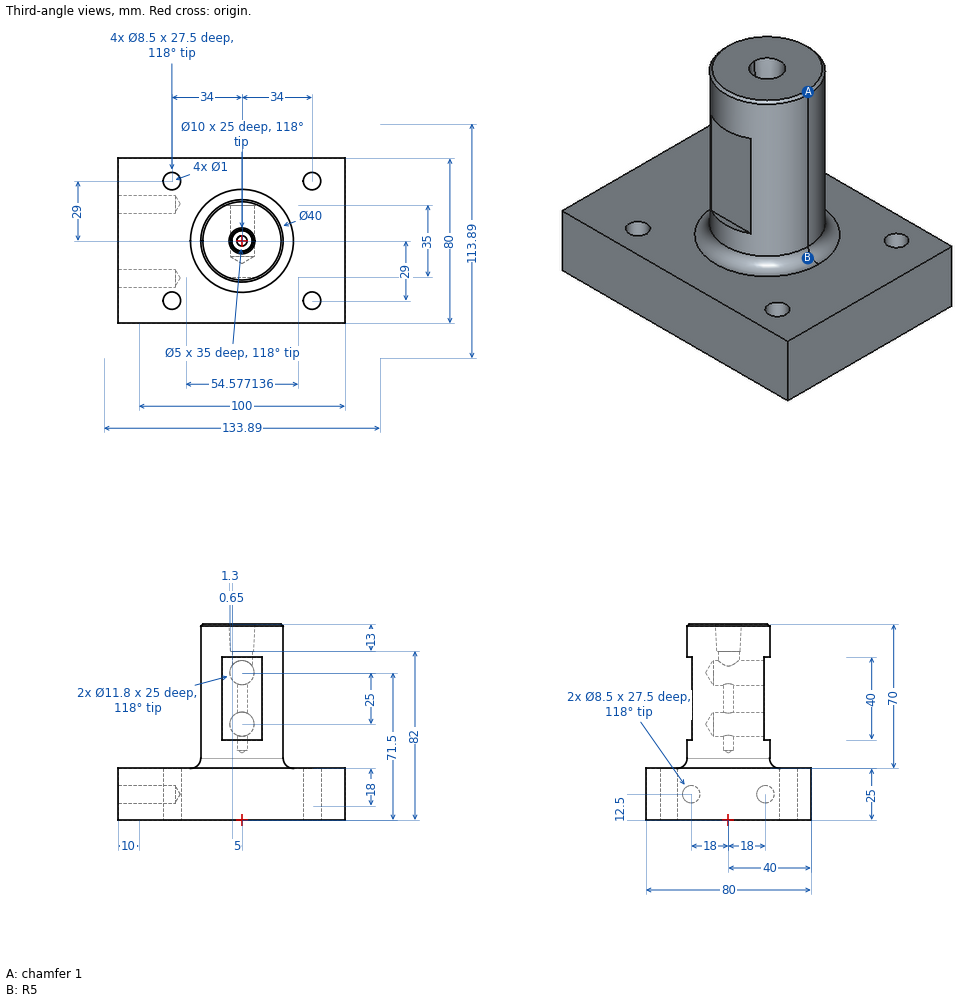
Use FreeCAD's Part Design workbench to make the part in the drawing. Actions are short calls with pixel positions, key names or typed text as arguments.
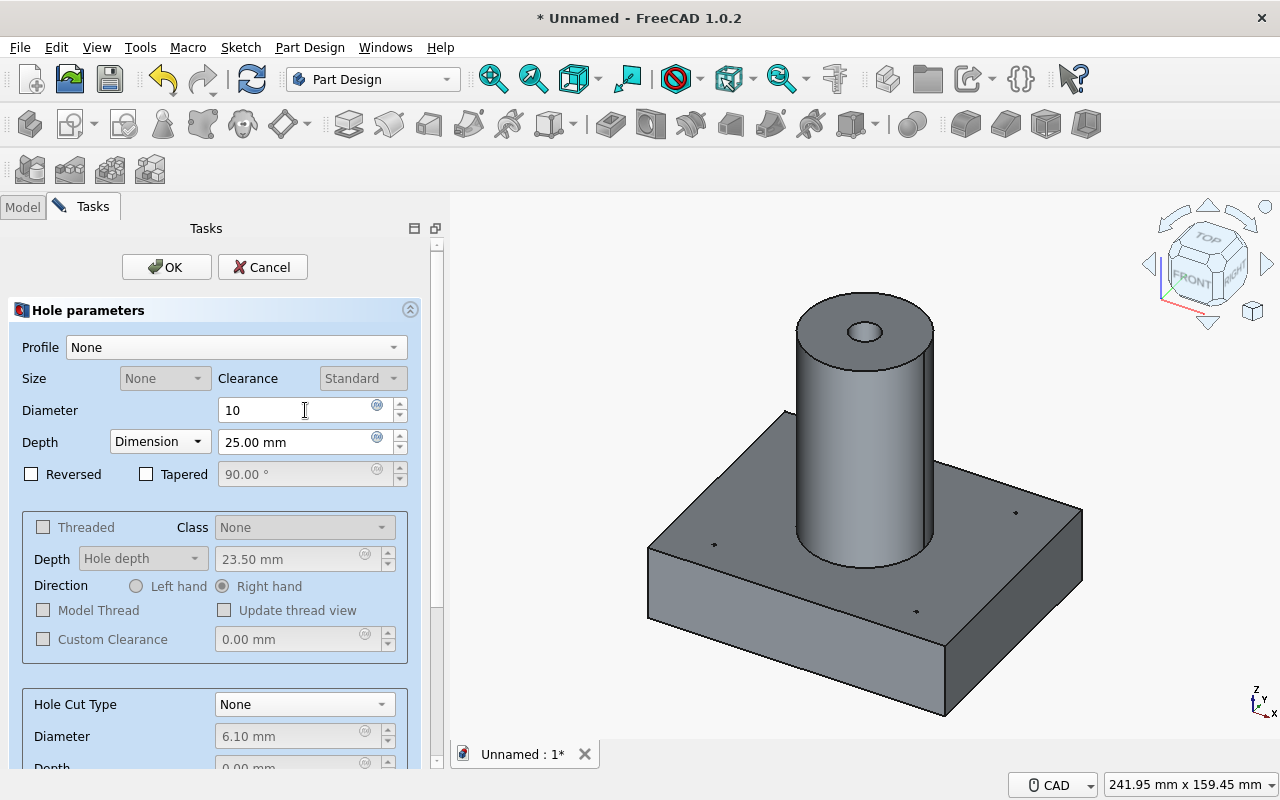
triple_click(305, 442)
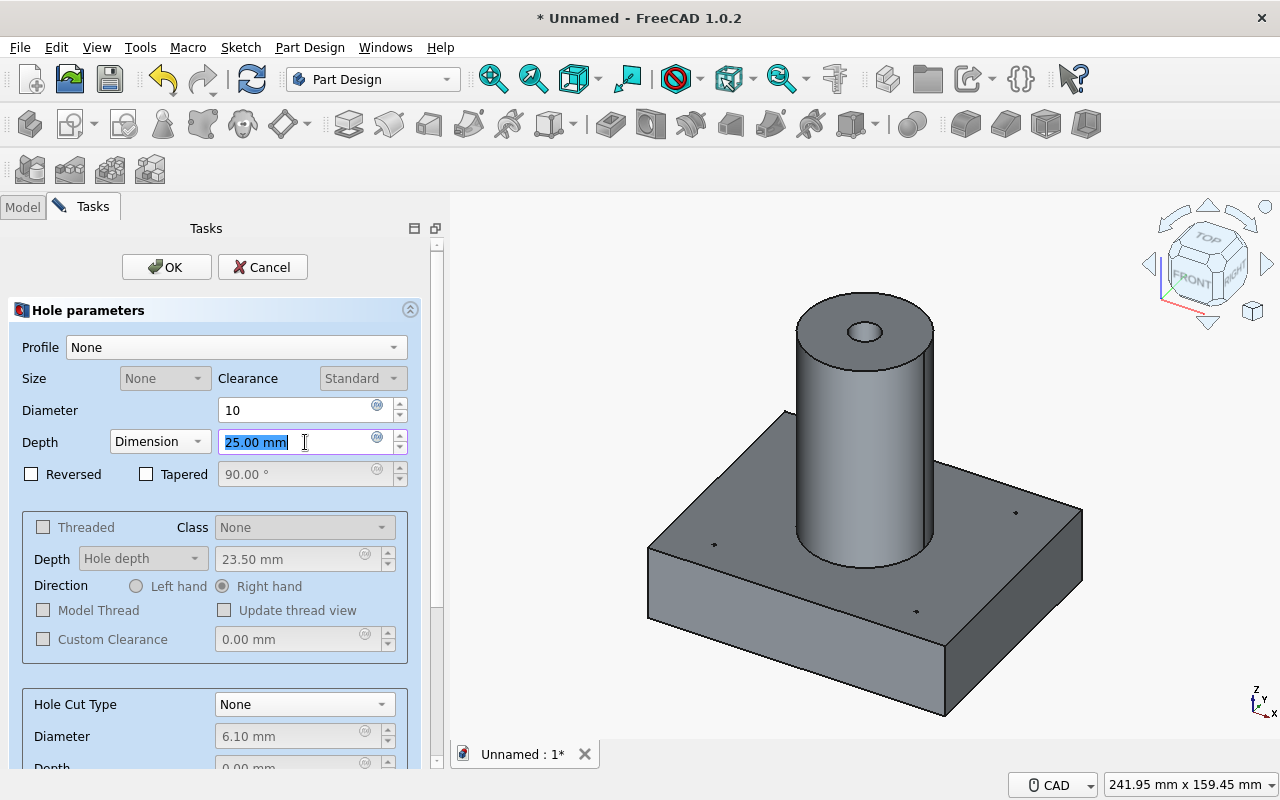
text(25)
key(Tab)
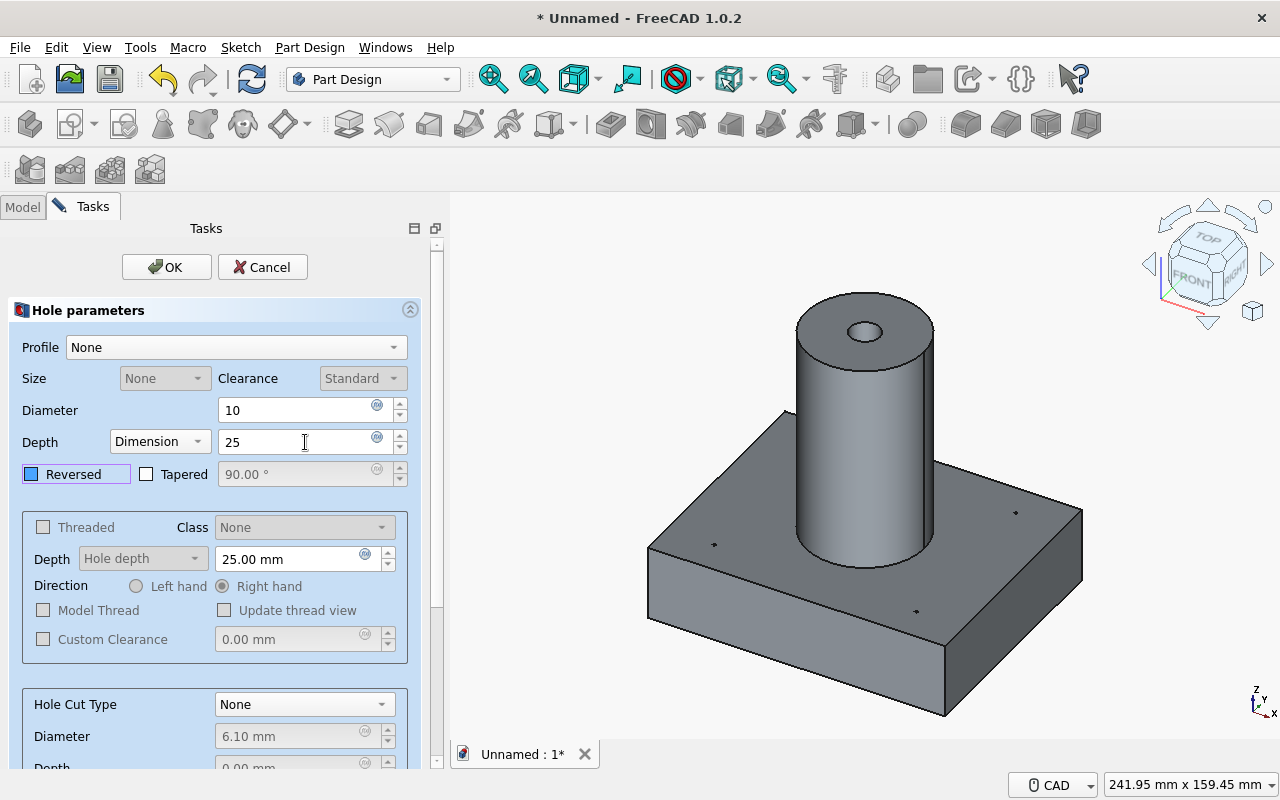
click(167, 267)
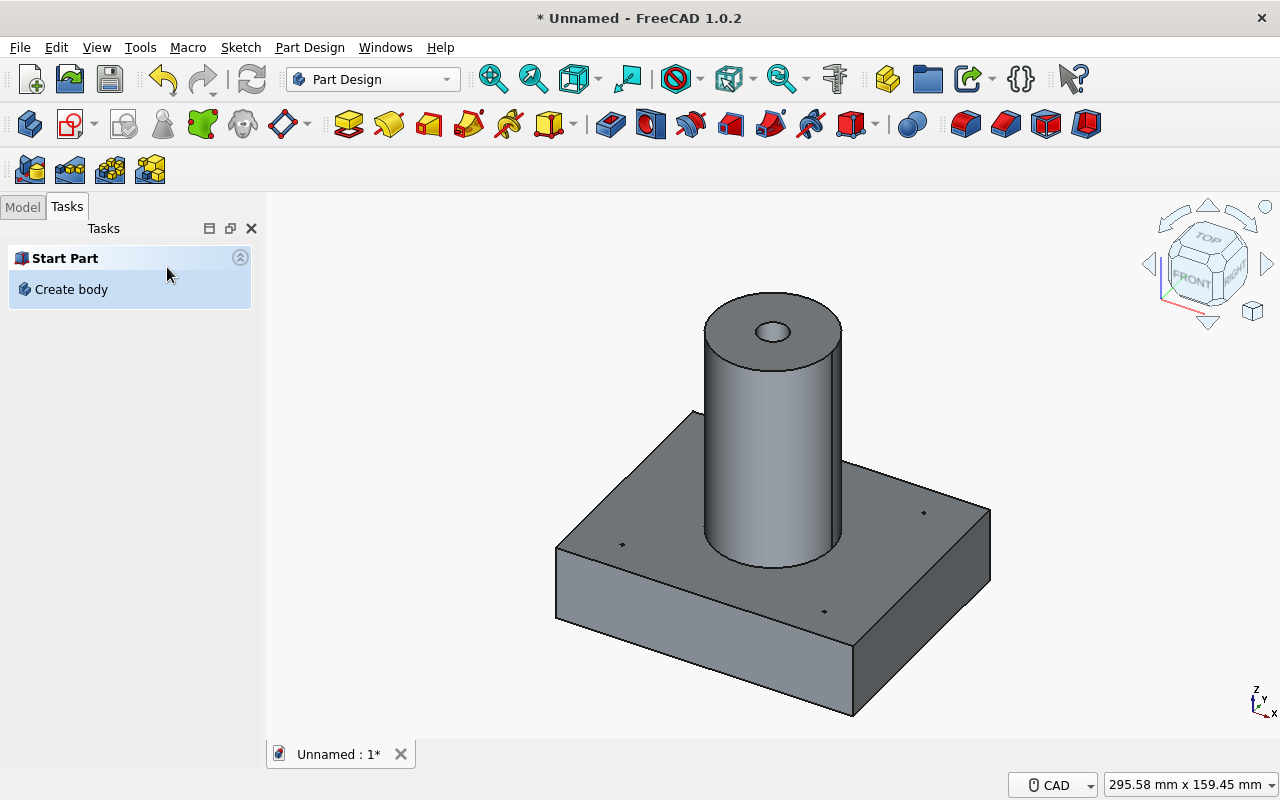
click(70, 124)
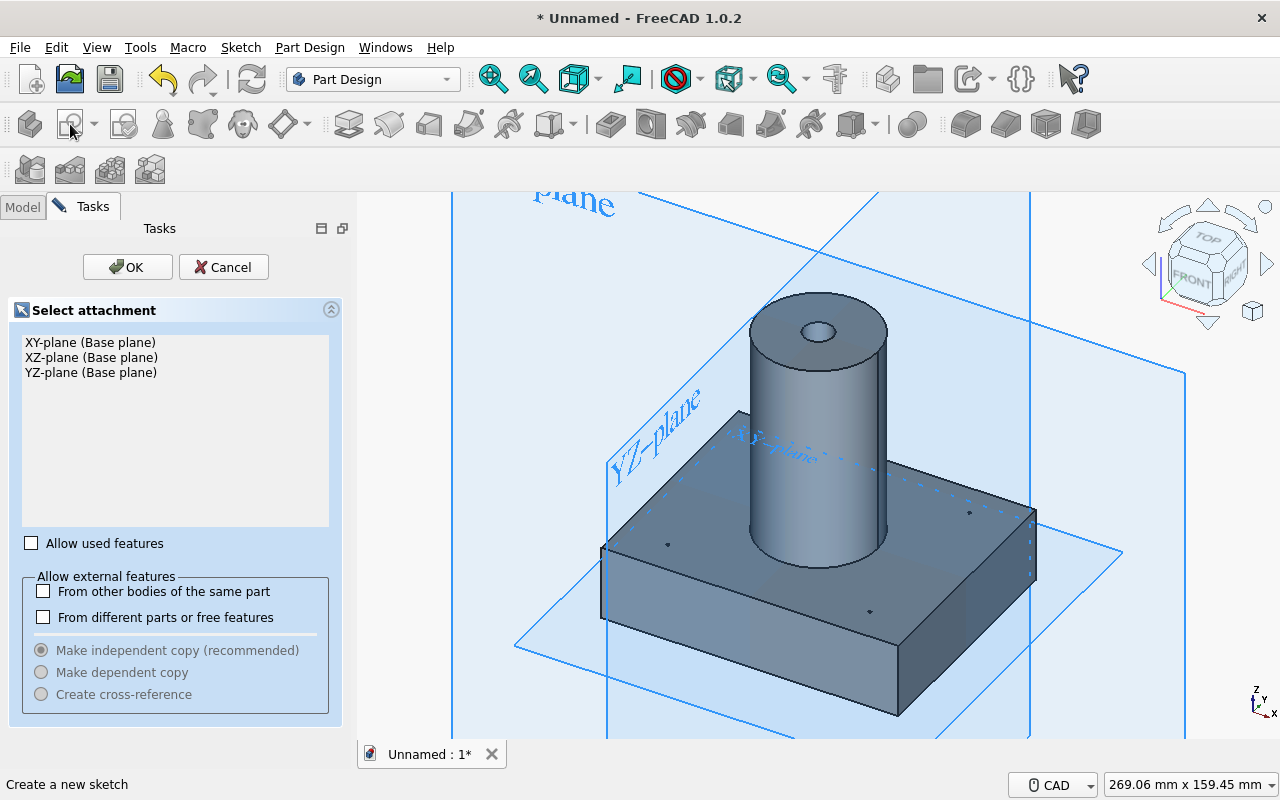
click(82, 358)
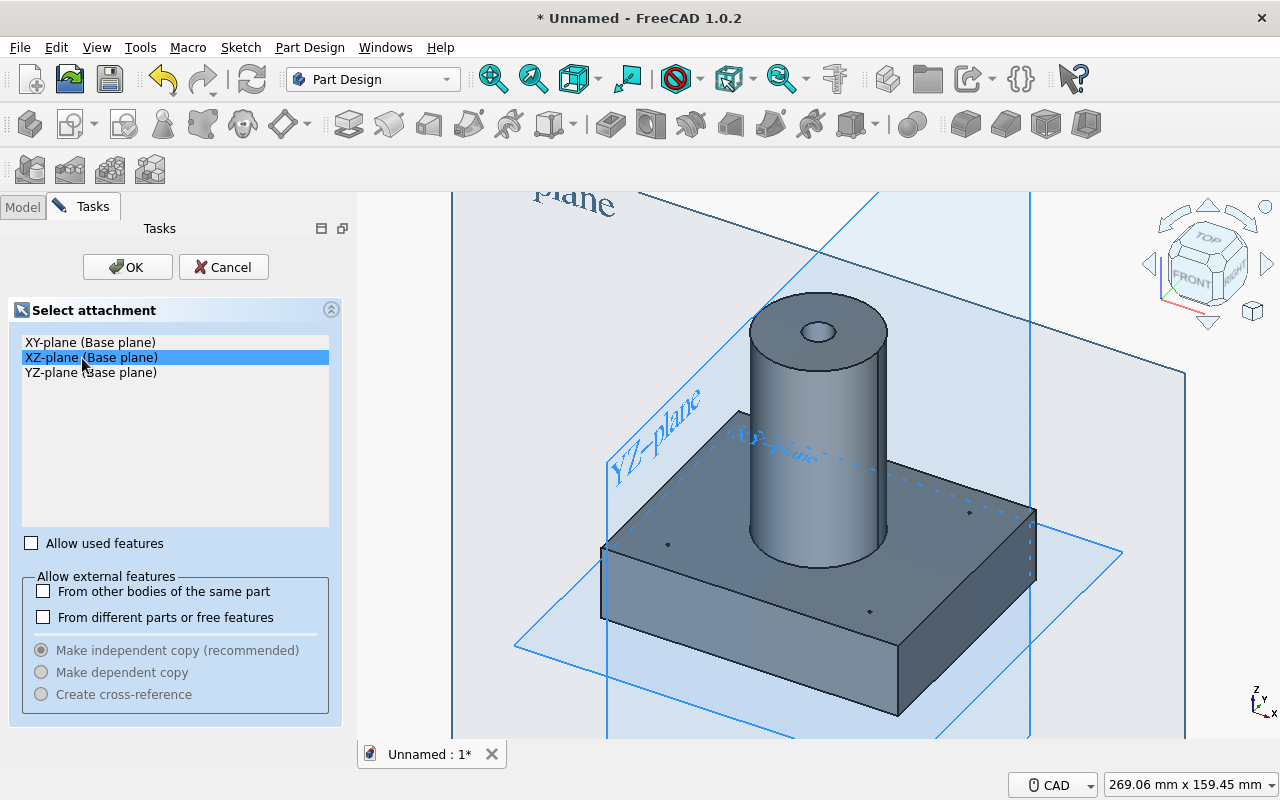
click(128, 267)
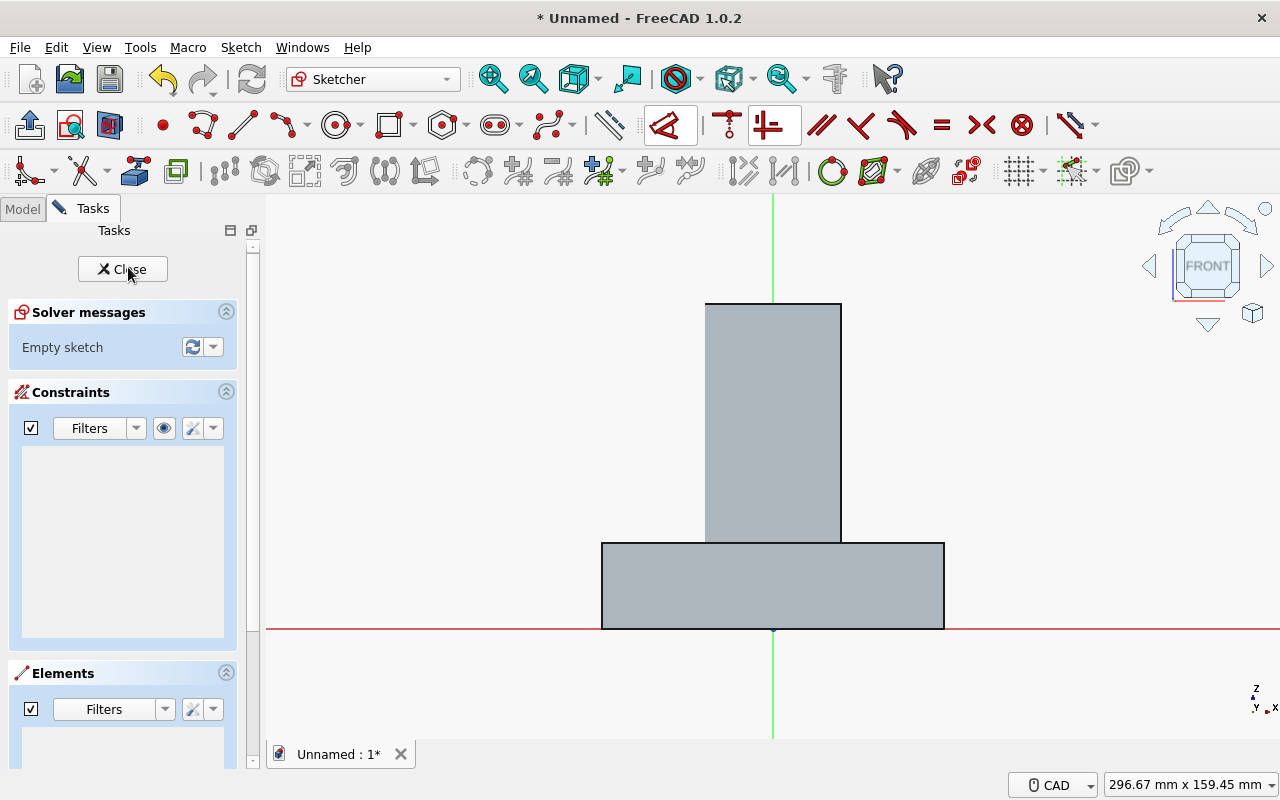
click(110, 126)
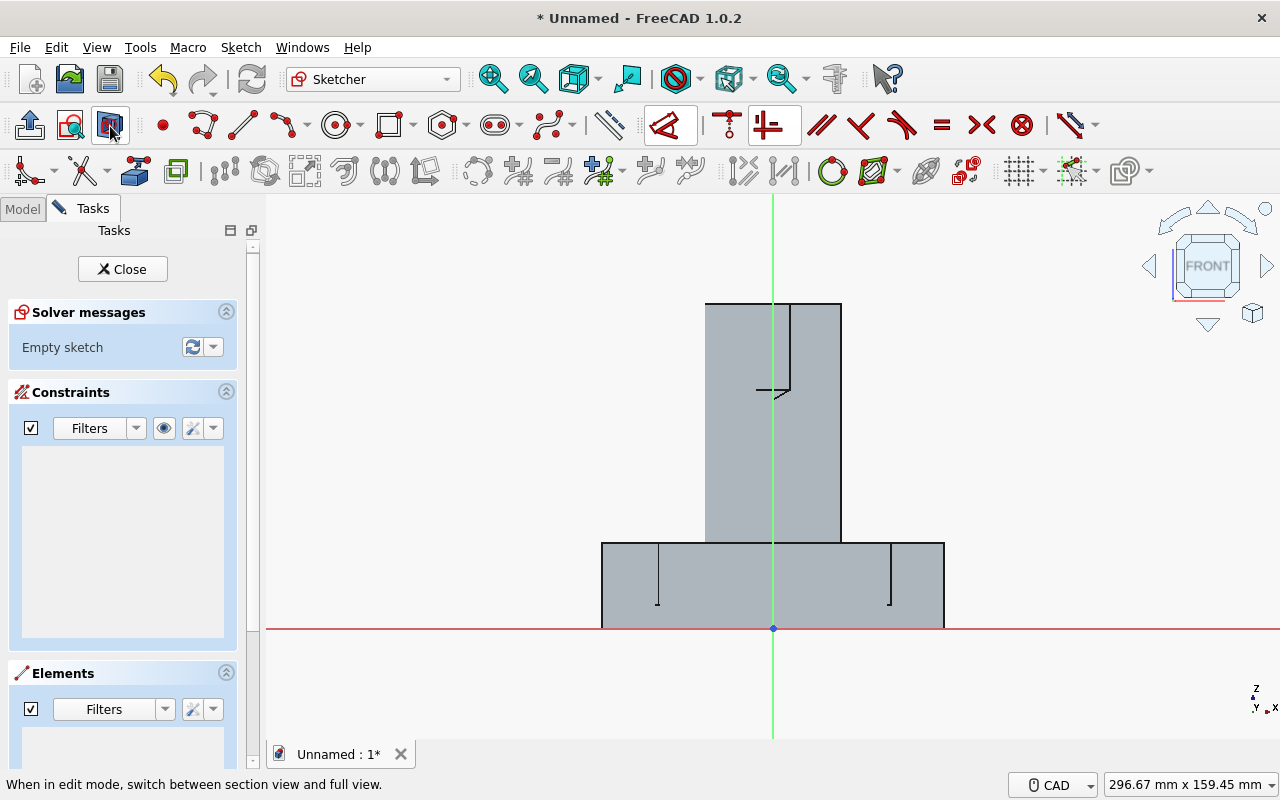
scroll(761, 304, up, 10)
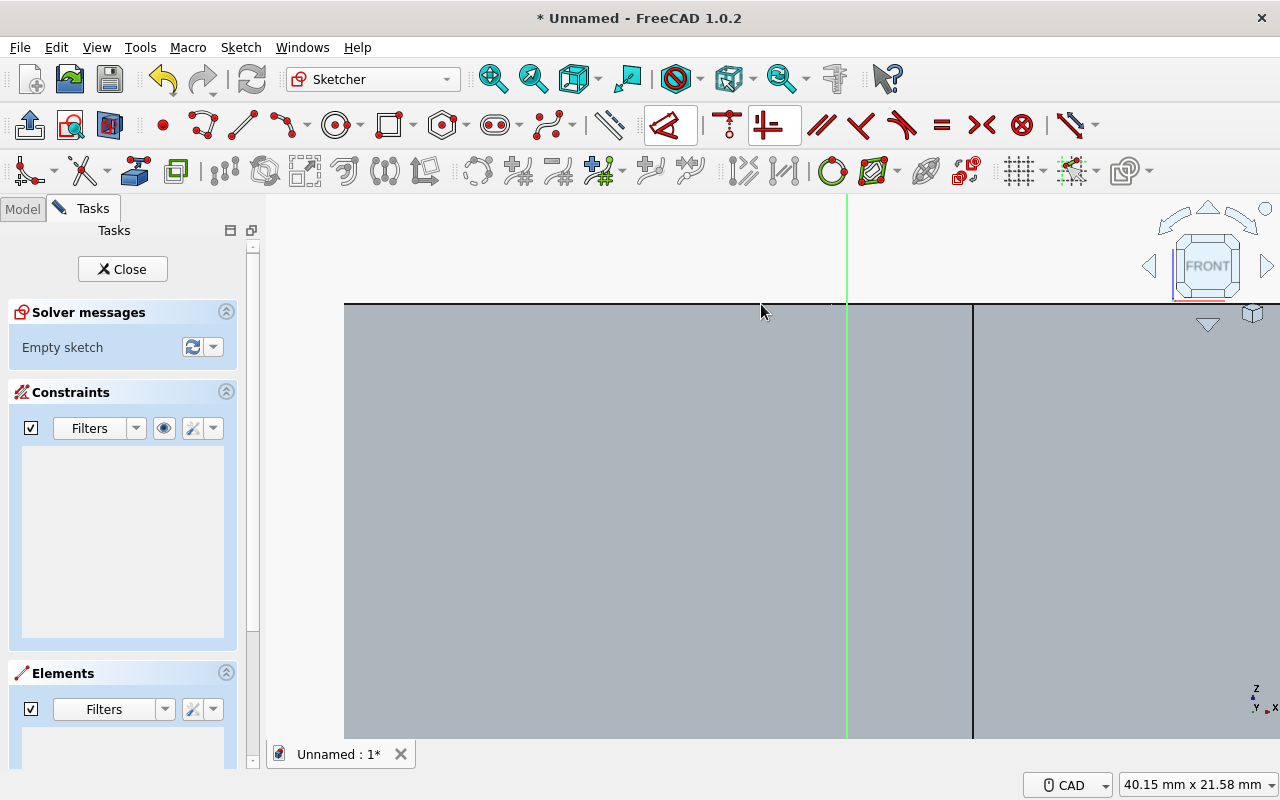
click(204, 126)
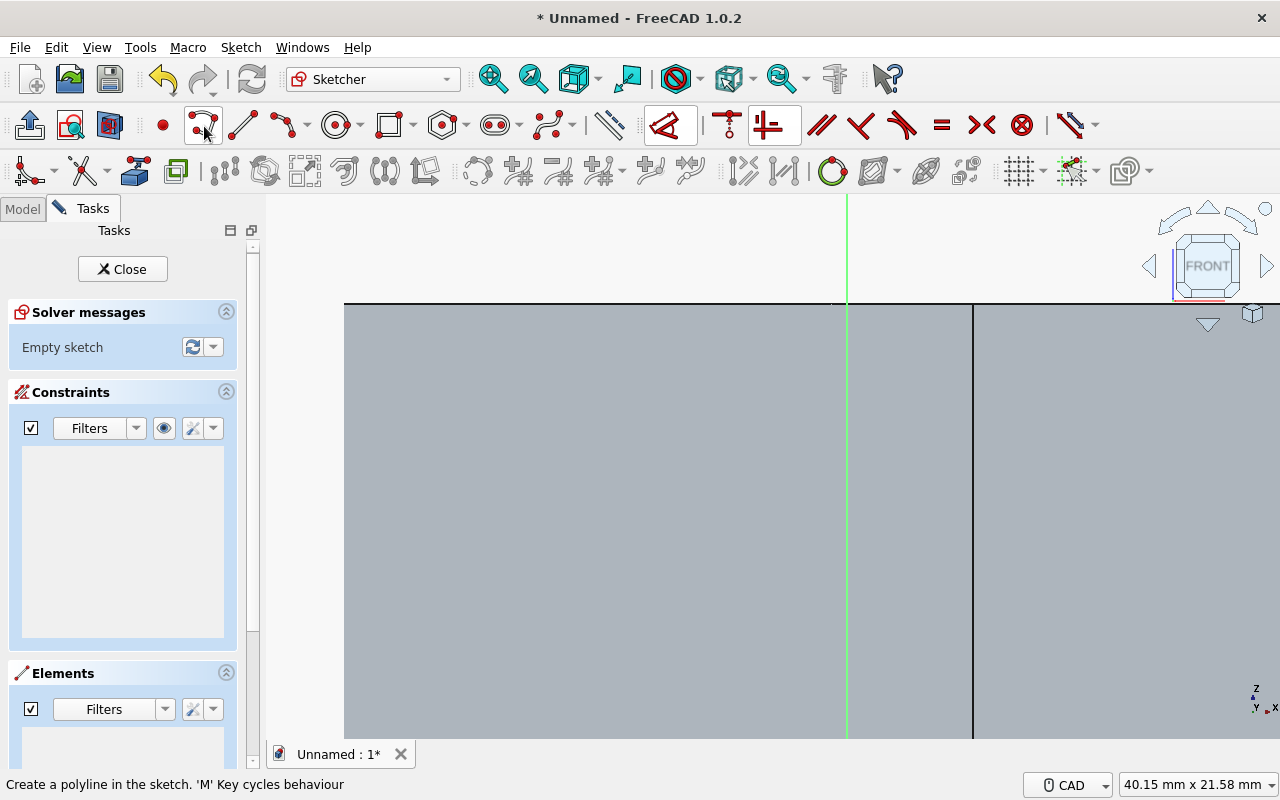
click(720, 632)
click(704, 632)
click(687, 304)
click(720, 304)